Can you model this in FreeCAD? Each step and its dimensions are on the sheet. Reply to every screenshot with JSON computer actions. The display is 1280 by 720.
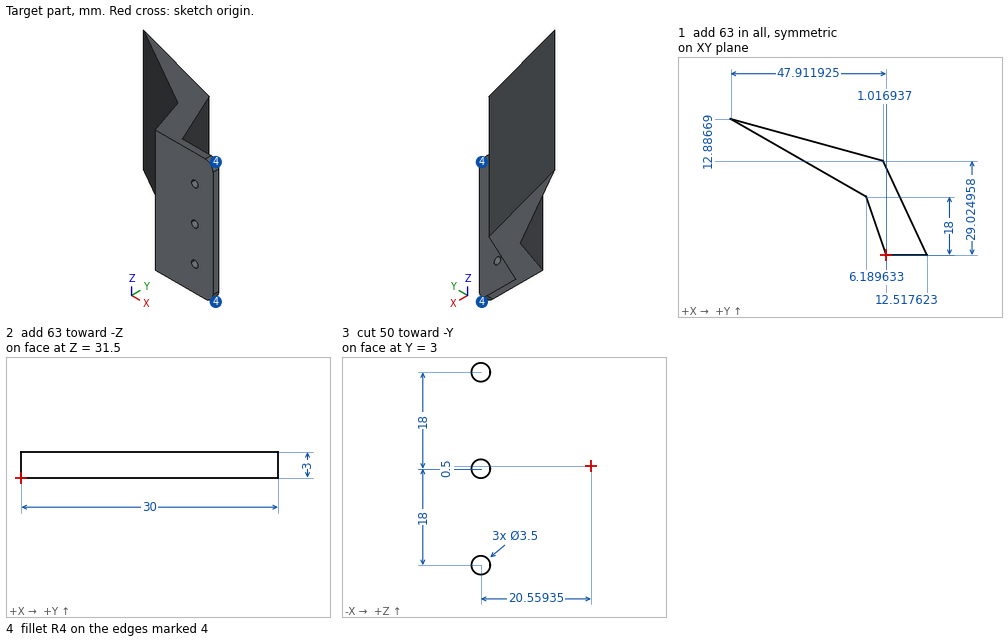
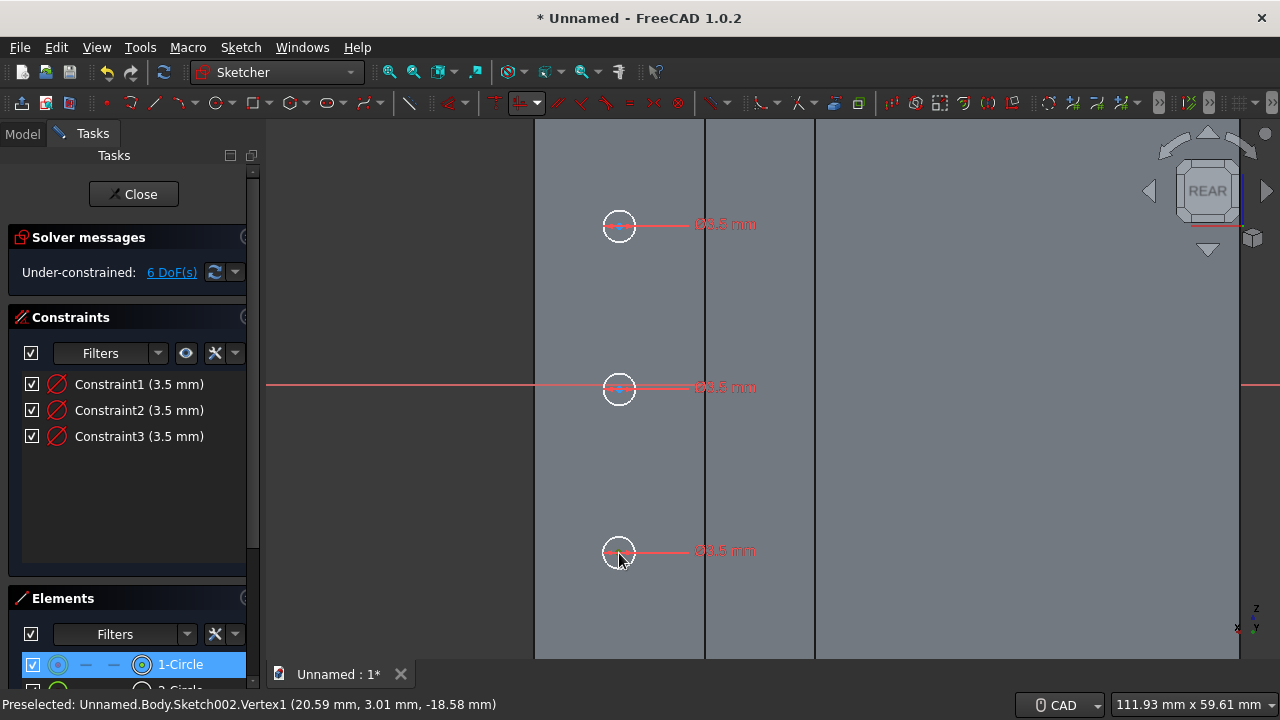
{"action": "left_click", "coordinate": [619, 389]}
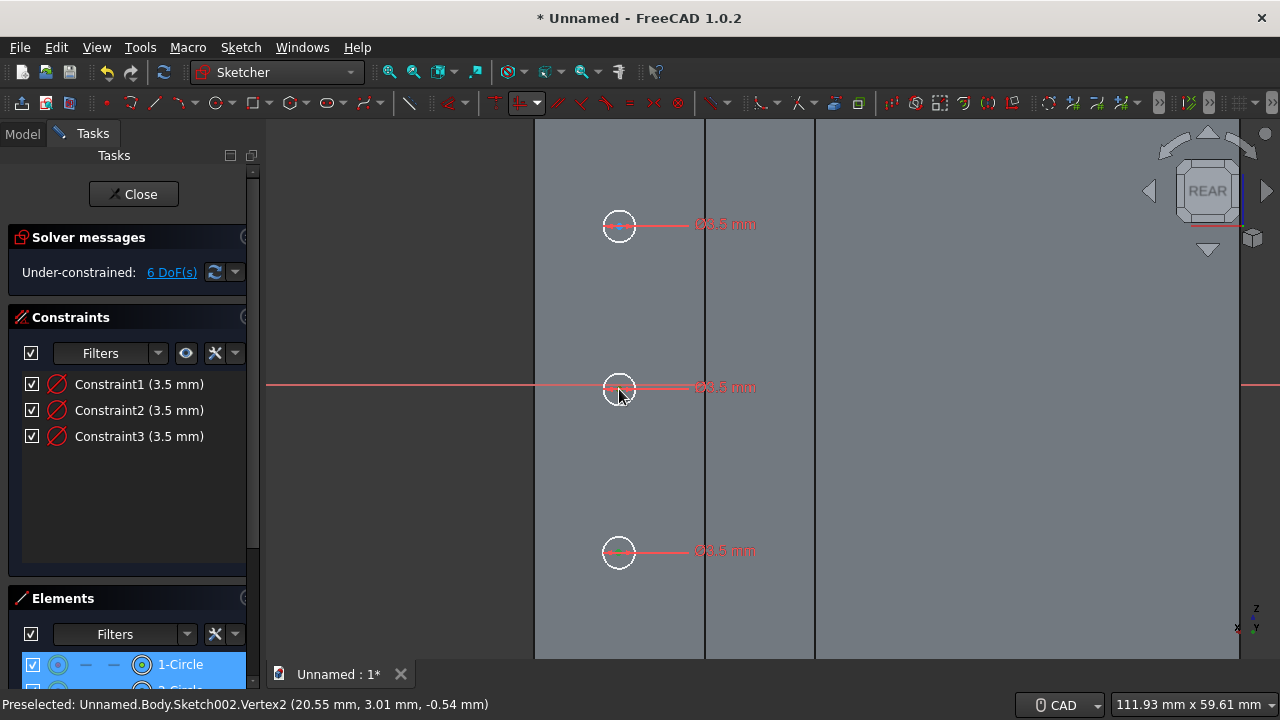
{"action": "key", "text": "v"}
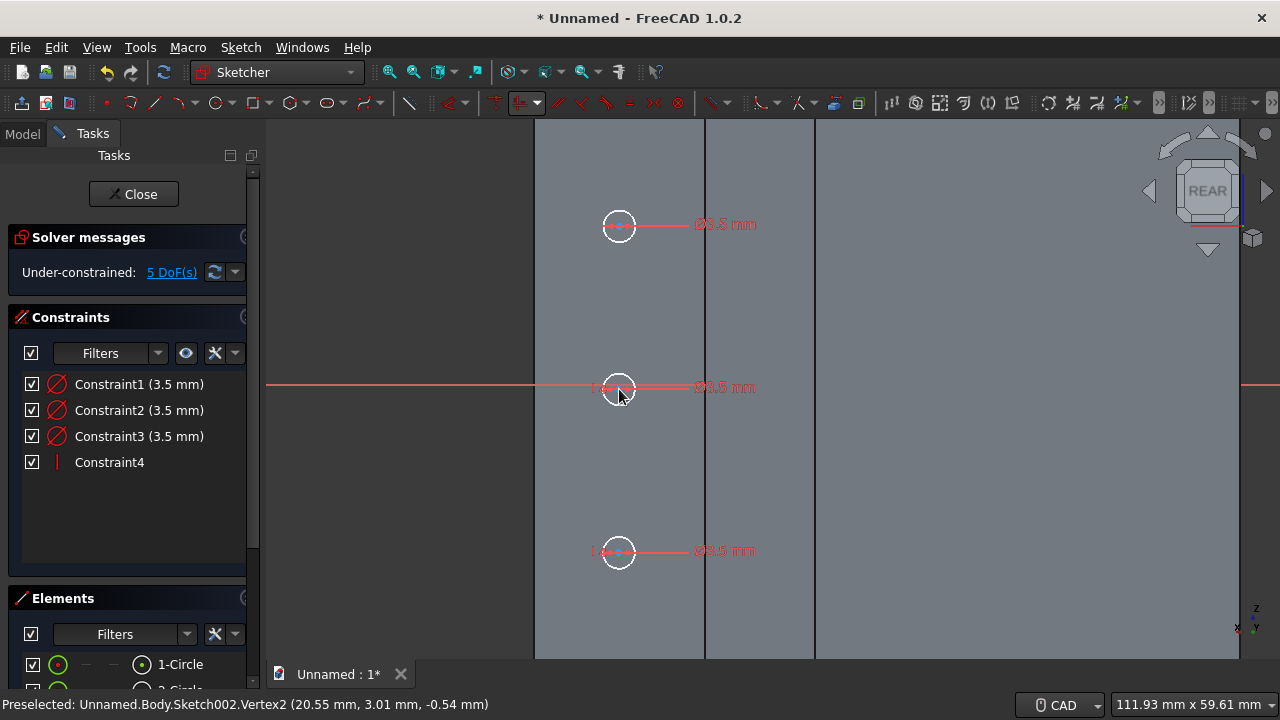
{"action": "left_click", "coordinate": [619, 389]}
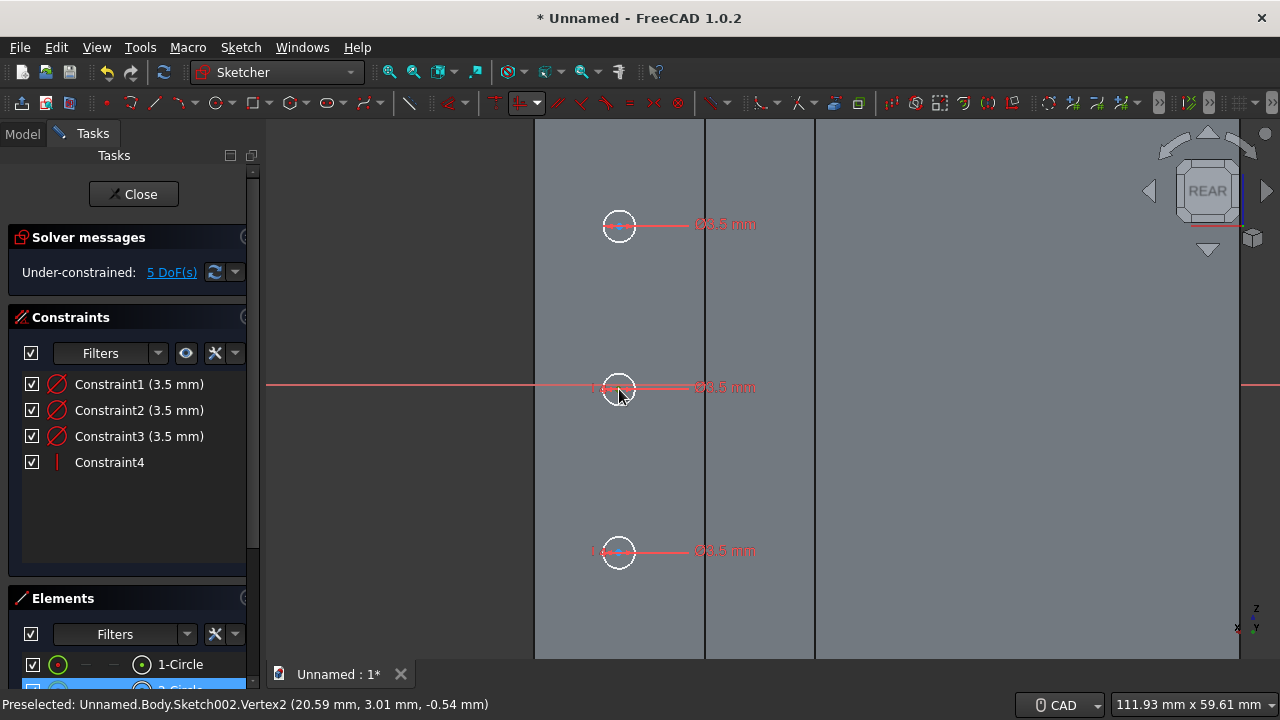
{"action": "left_click", "coordinate": [619, 226]}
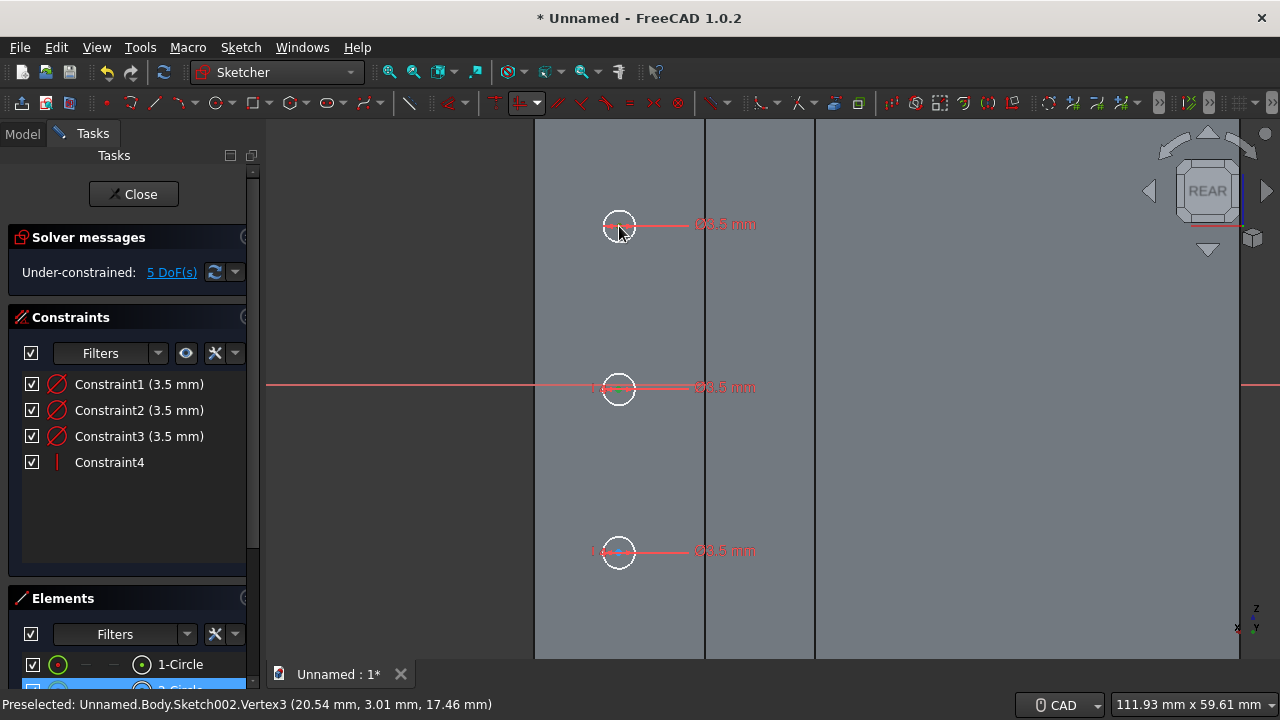
{"action": "key", "text": "v"}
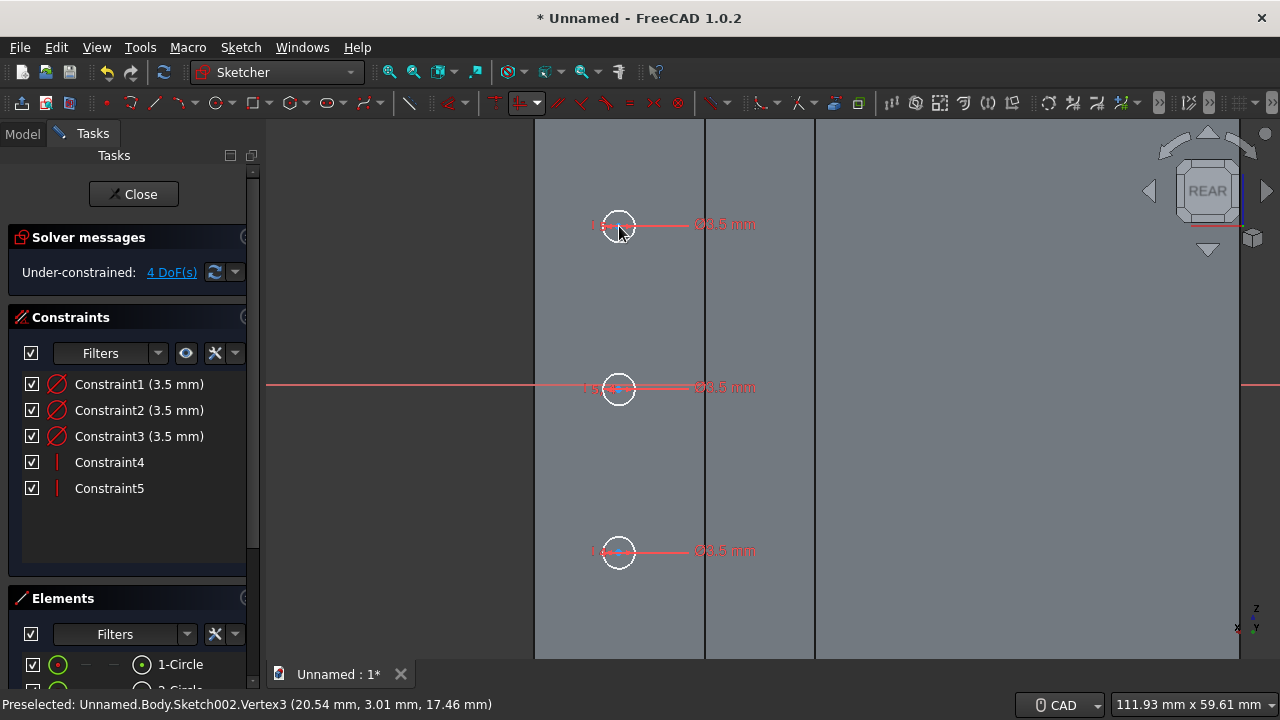
{"action": "left_click", "coordinate": [448, 104]}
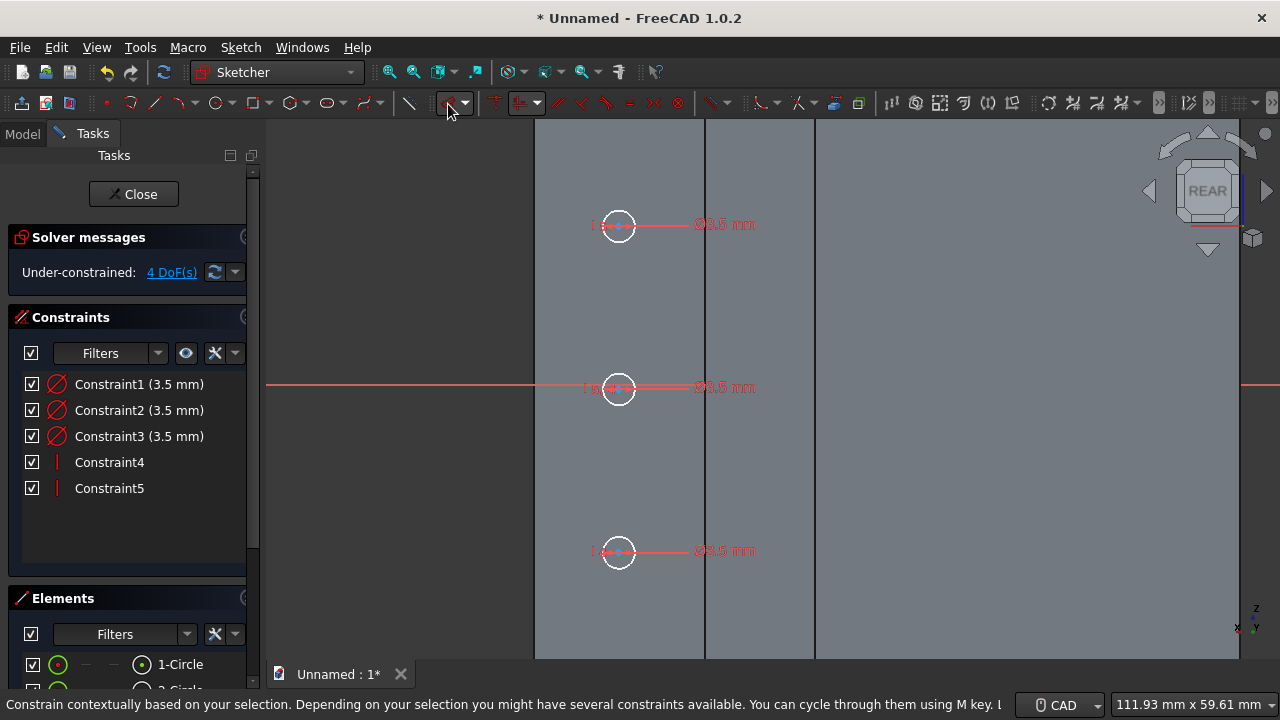
{"action": "scroll", "coordinate": [619, 389], "scroll_direction": "up", "scroll_amount": 11}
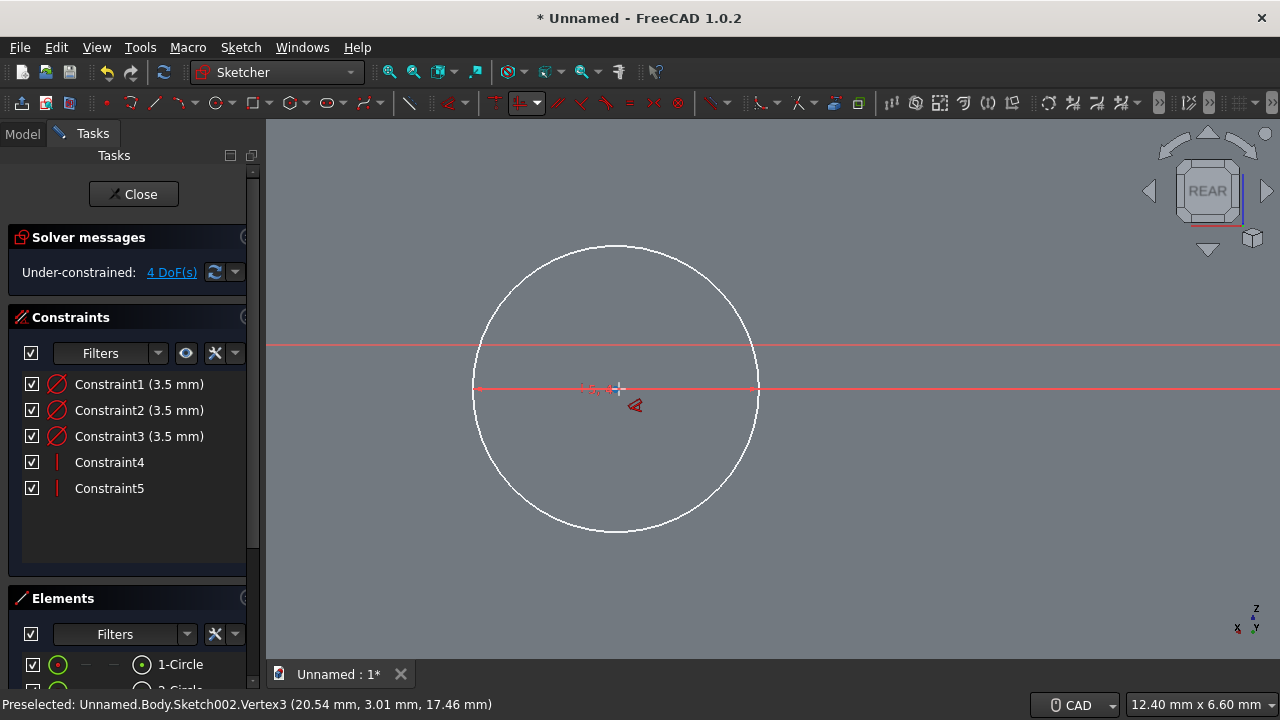
{"action": "left_click", "coordinate": [616, 389]}
{"action": "left_click", "coordinate": [582, 367]}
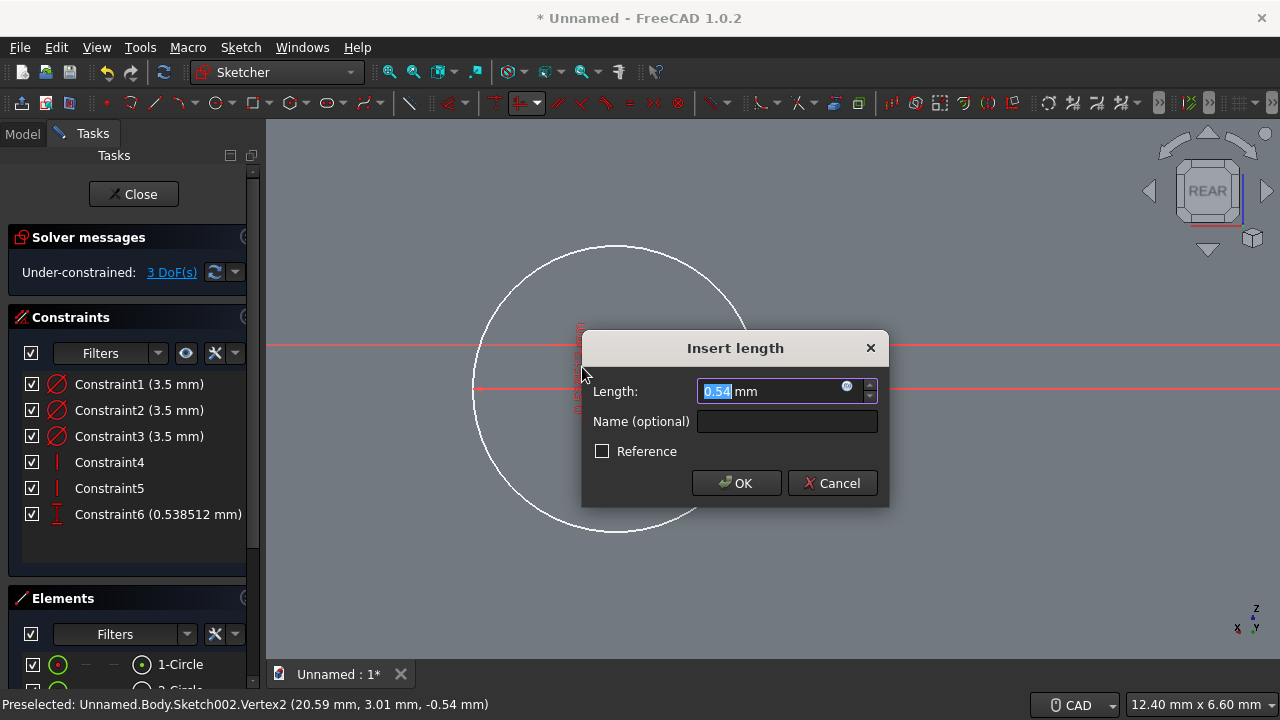
{"action": "type", "text": "0.5"}
{"action": "key", "text": "Return"}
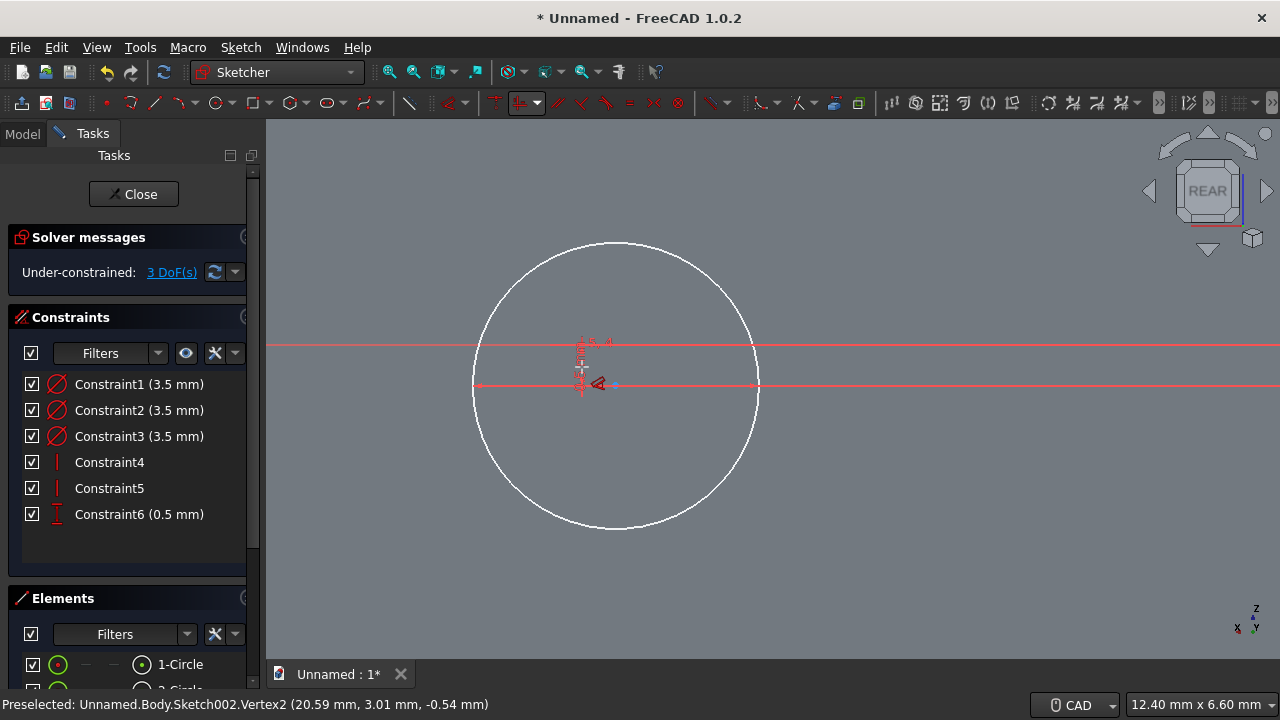
{"action": "scroll", "coordinate": [619, 389], "scroll_direction": "down", "scroll_amount": 11}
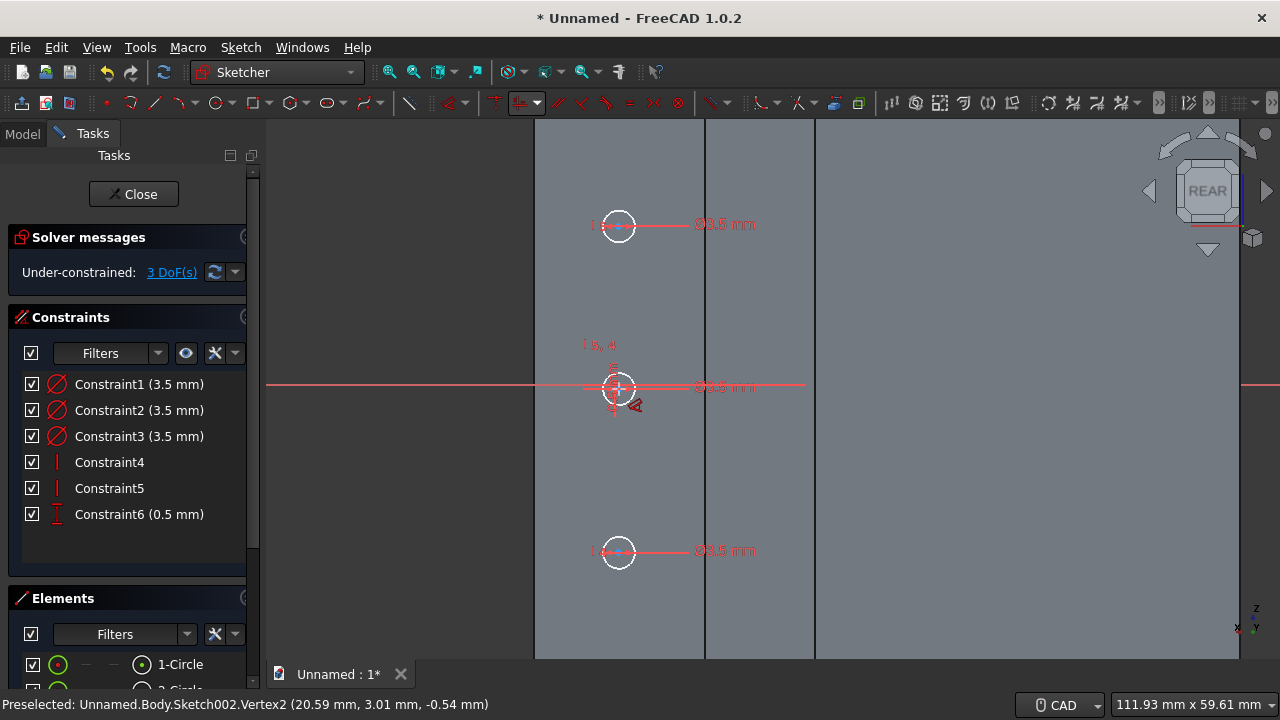
{"action": "left_click", "coordinate": [619, 553]}